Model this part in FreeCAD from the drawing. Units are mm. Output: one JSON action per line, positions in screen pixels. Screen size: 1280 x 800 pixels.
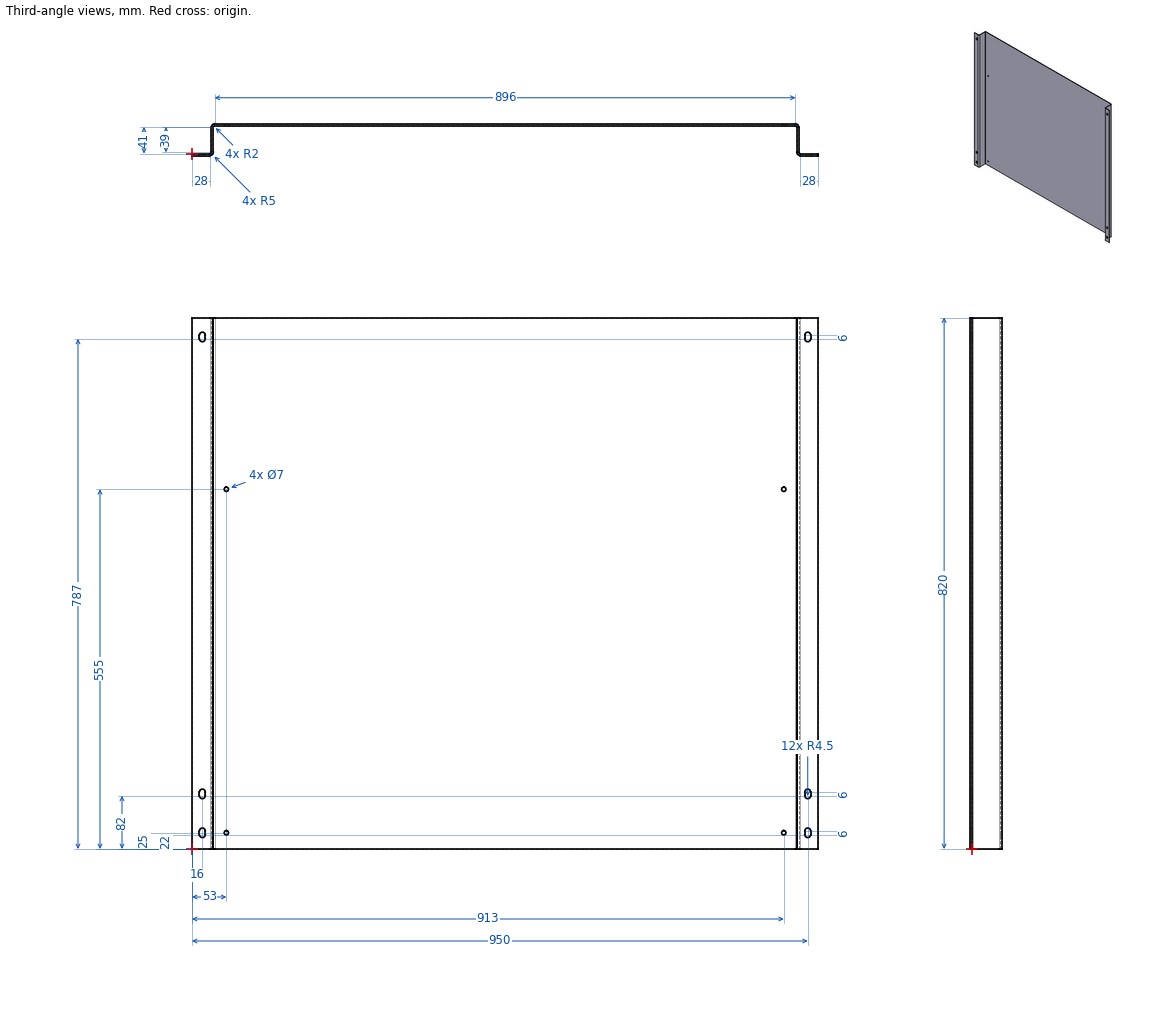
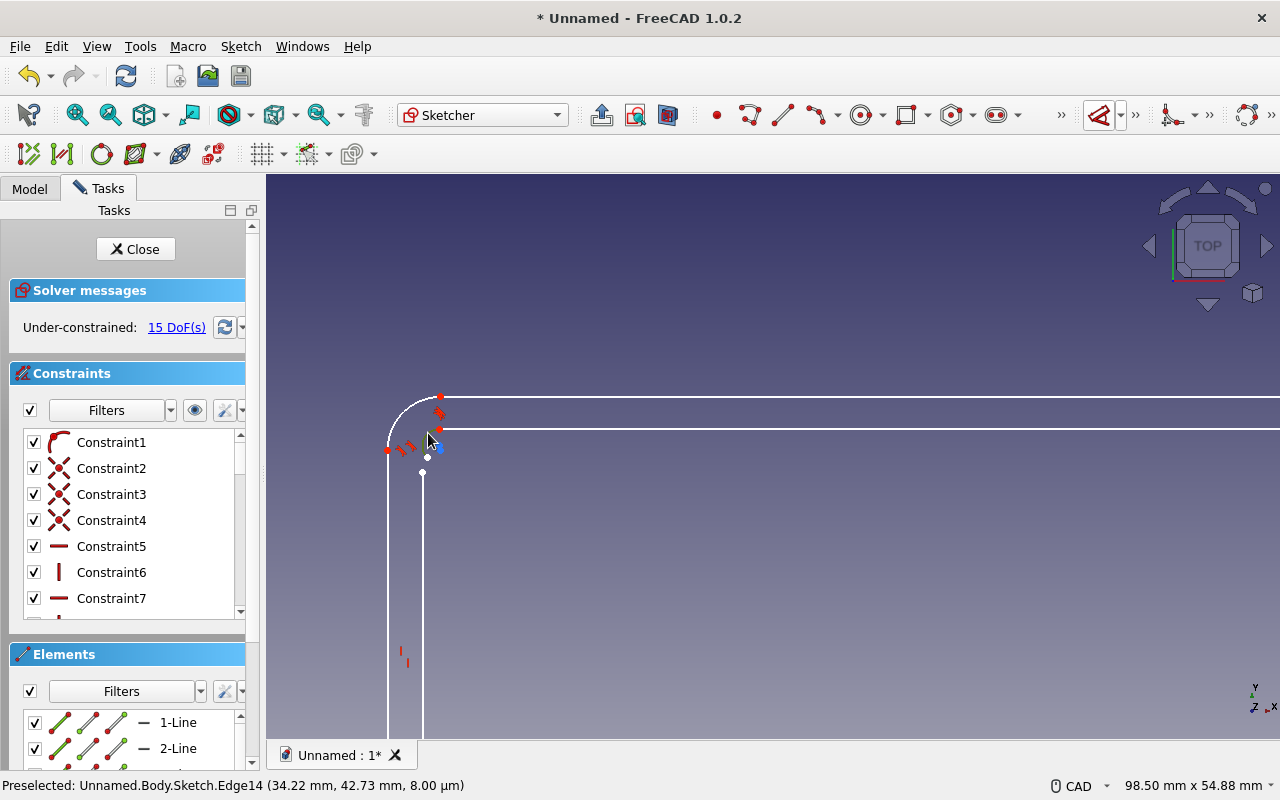
{"action": "left_click", "coordinate": [417, 403]}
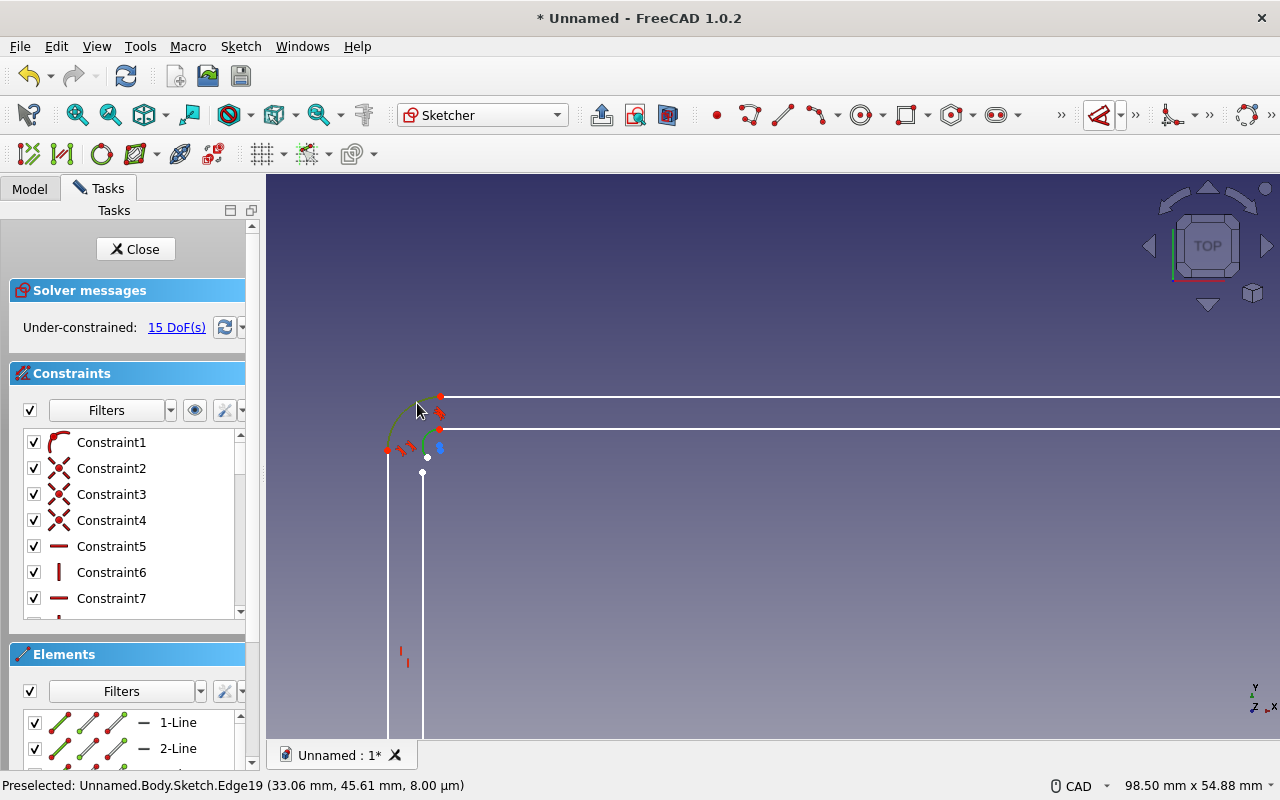
{"action": "key", "text": "c"}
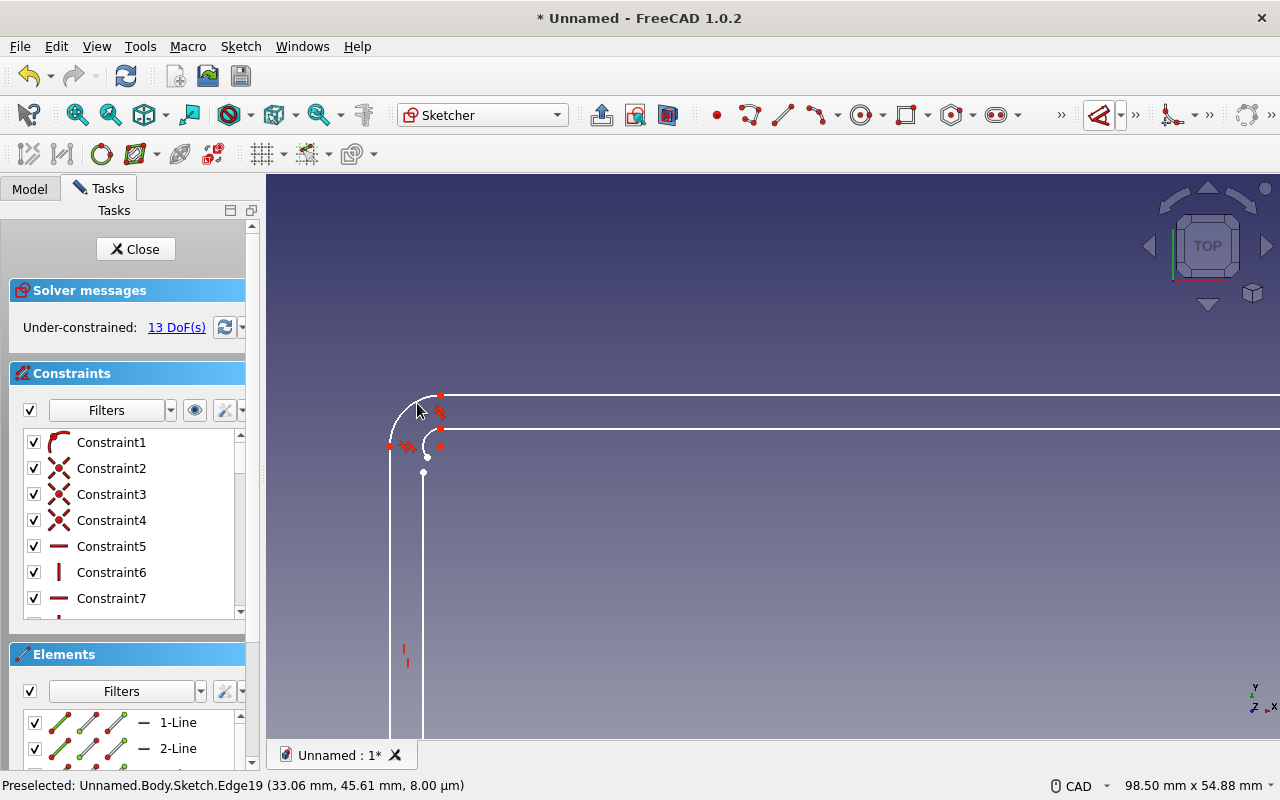
{"action": "scroll", "coordinate": [423, 444], "scroll_direction": "down", "scroll_amount": 14}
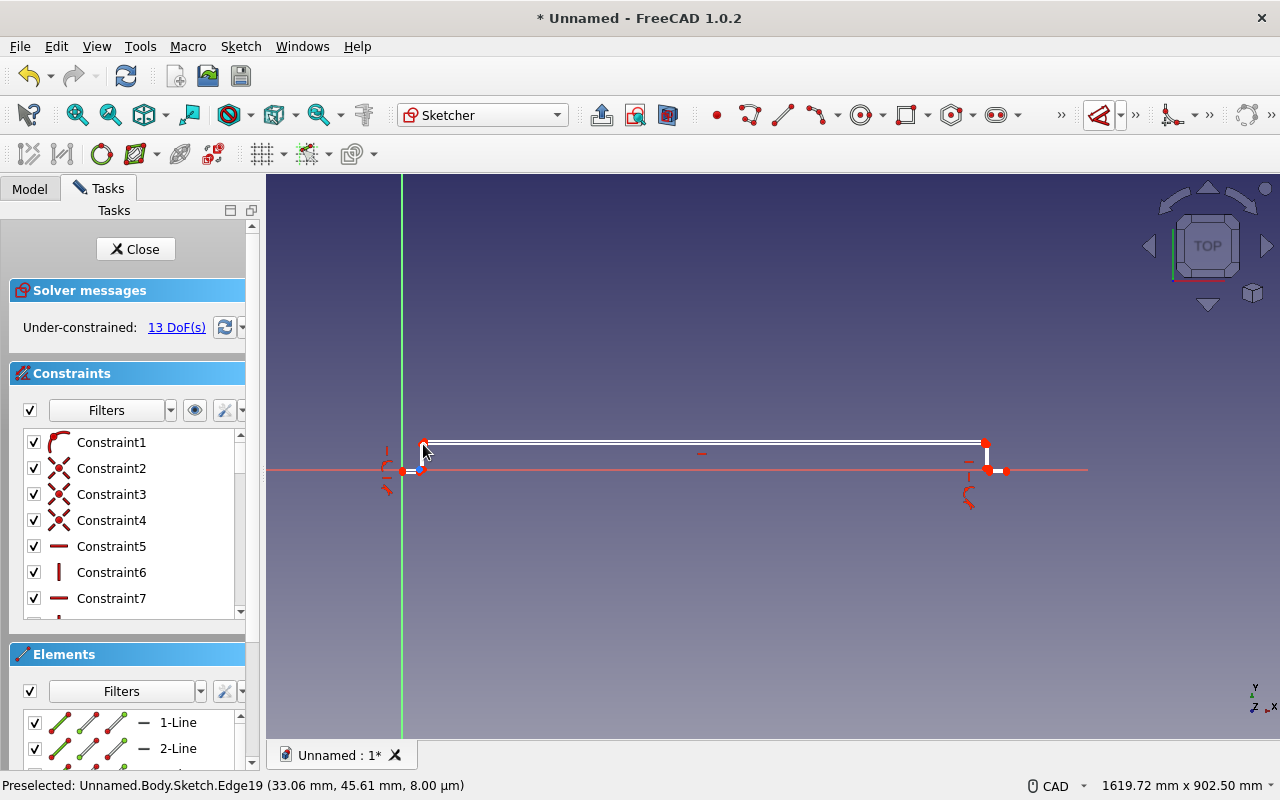
{"action": "scroll", "coordinate": [421, 472], "scroll_direction": "up", "scroll_amount": 11}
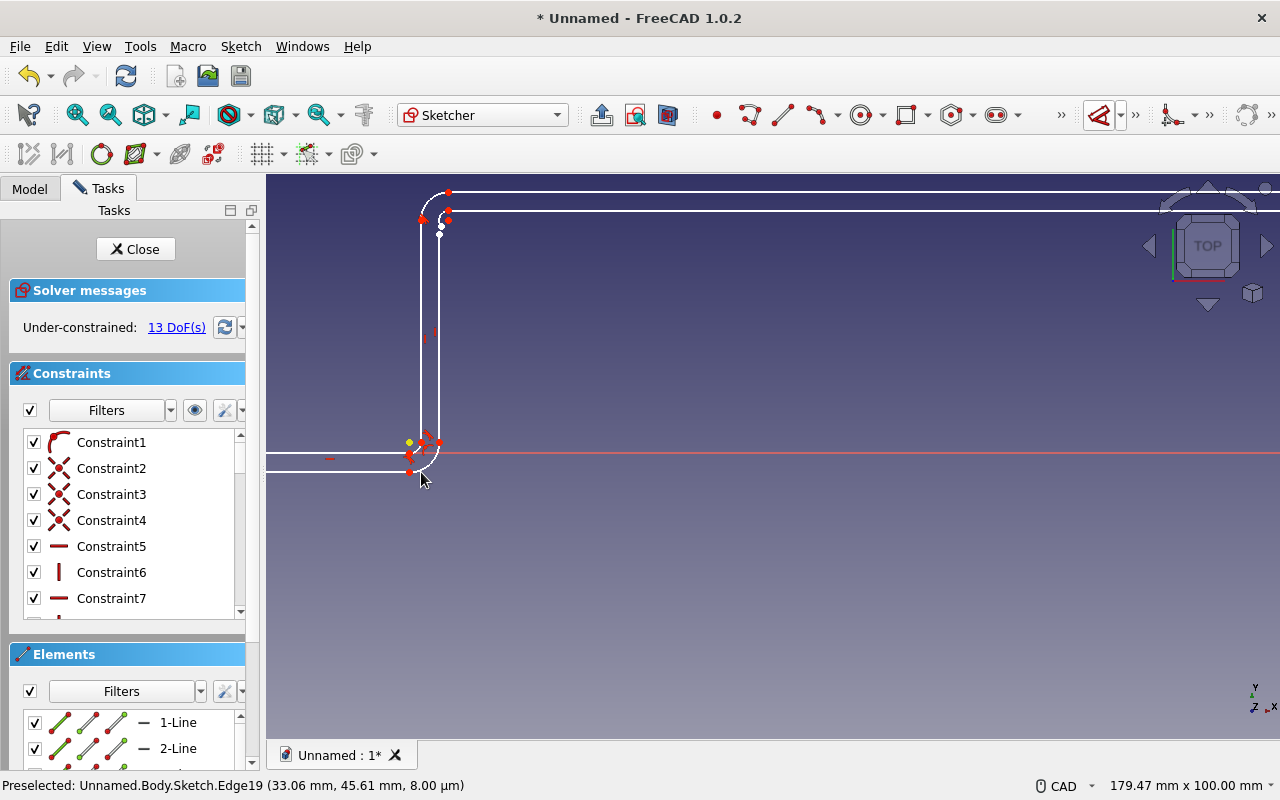
{"action": "left_click", "coordinate": [423, 469]}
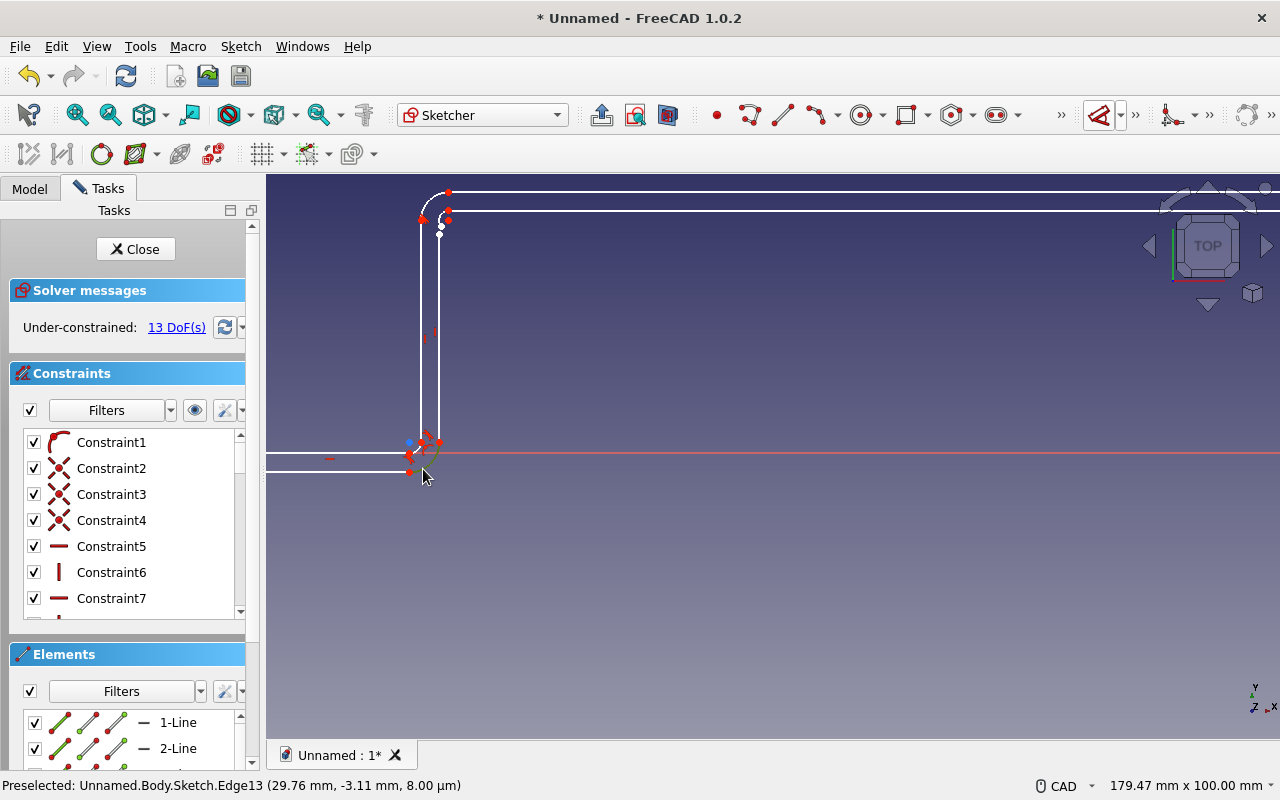
{"action": "scroll", "coordinate": [418, 450], "scroll_direction": "up", "scroll_amount": 3}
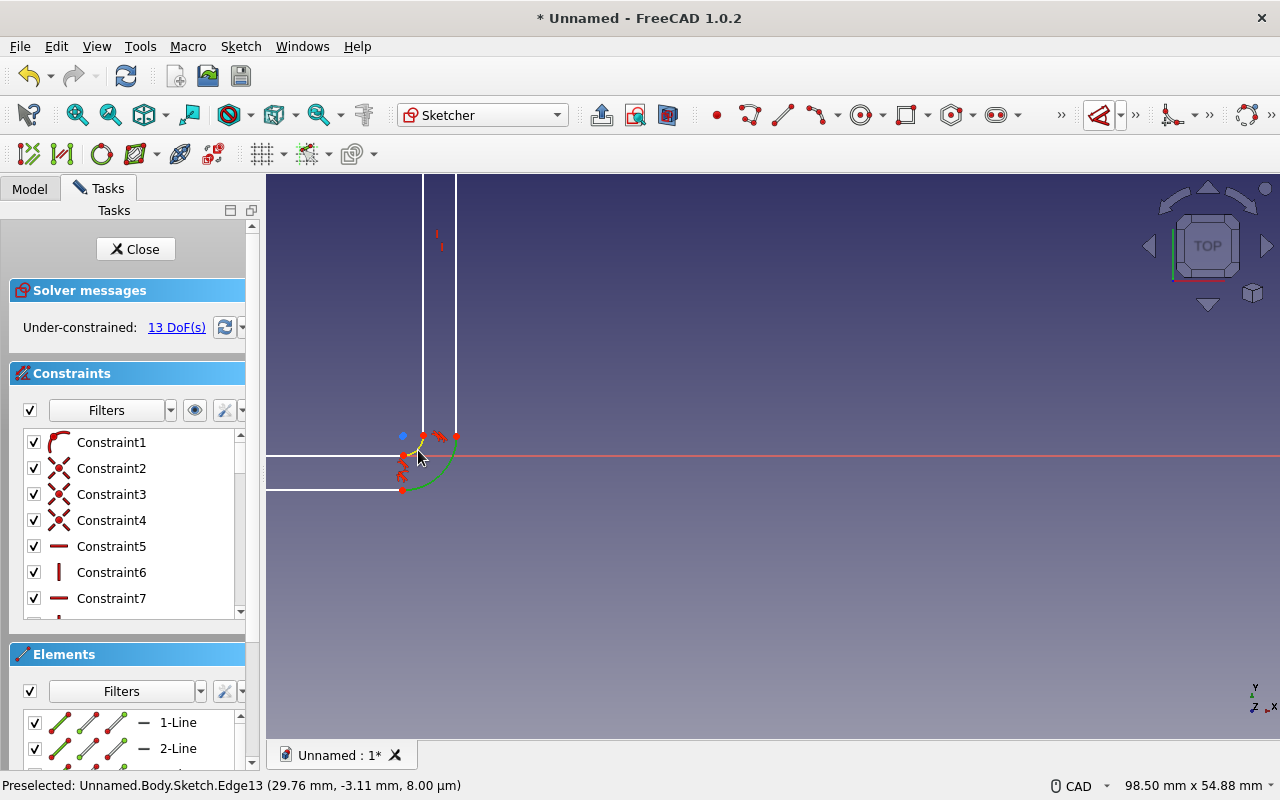
{"action": "left_click", "coordinate": [417, 450]}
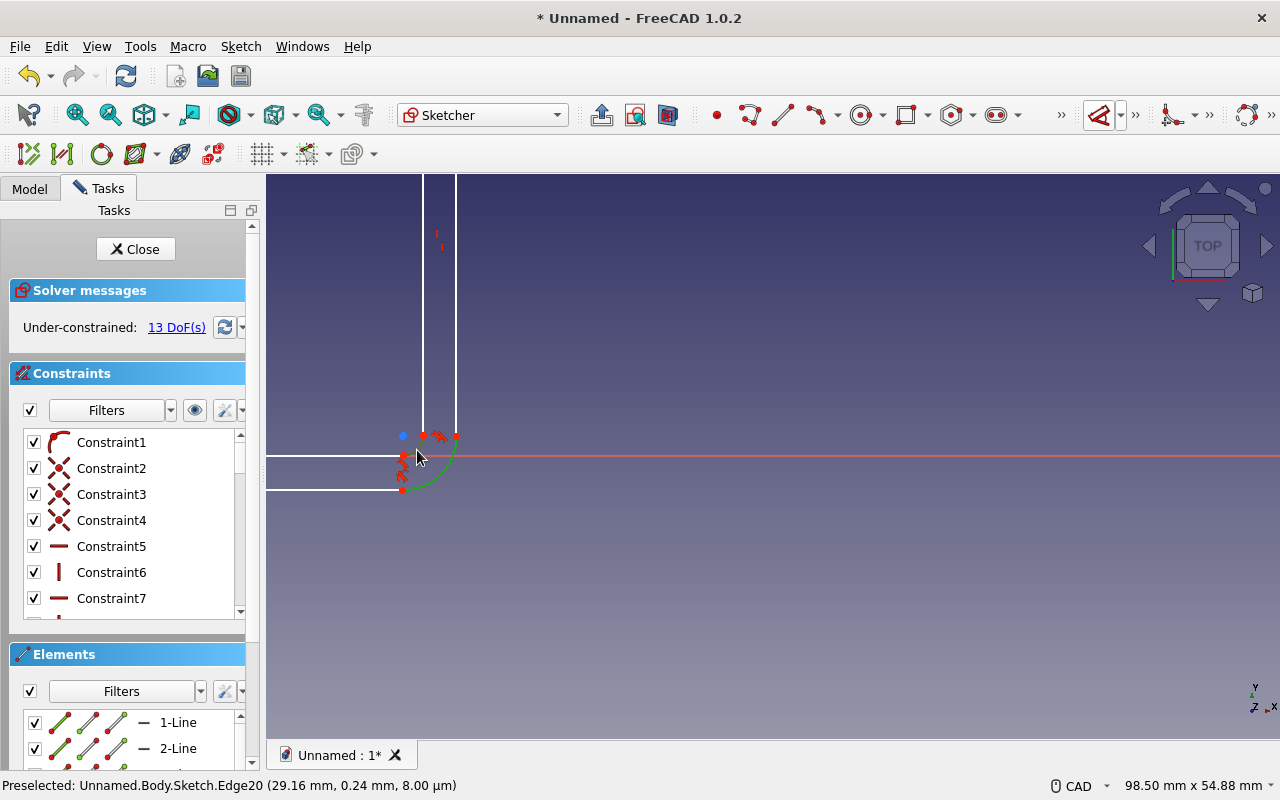
{"action": "key", "text": "c"}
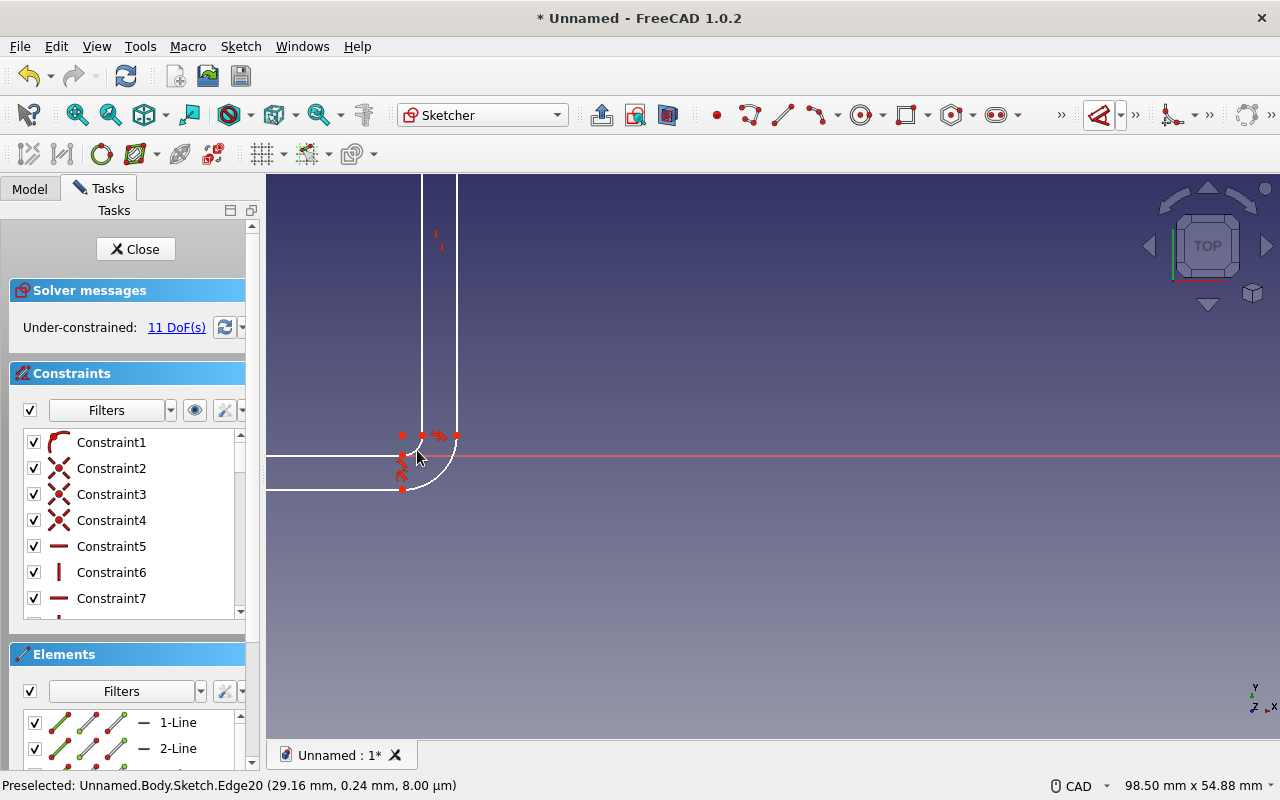
{"action": "scroll", "coordinate": [421, 471], "scroll_direction": "down", "scroll_amount": 14}